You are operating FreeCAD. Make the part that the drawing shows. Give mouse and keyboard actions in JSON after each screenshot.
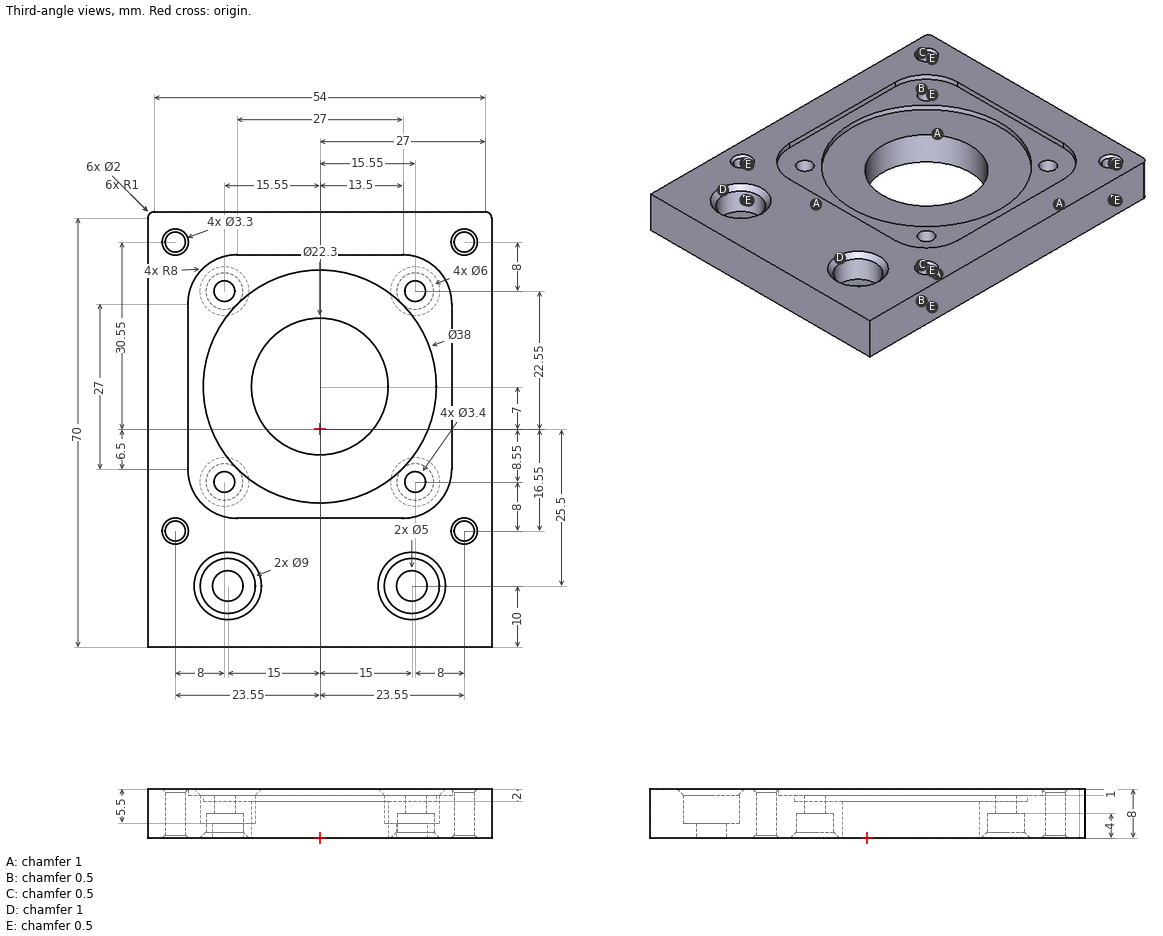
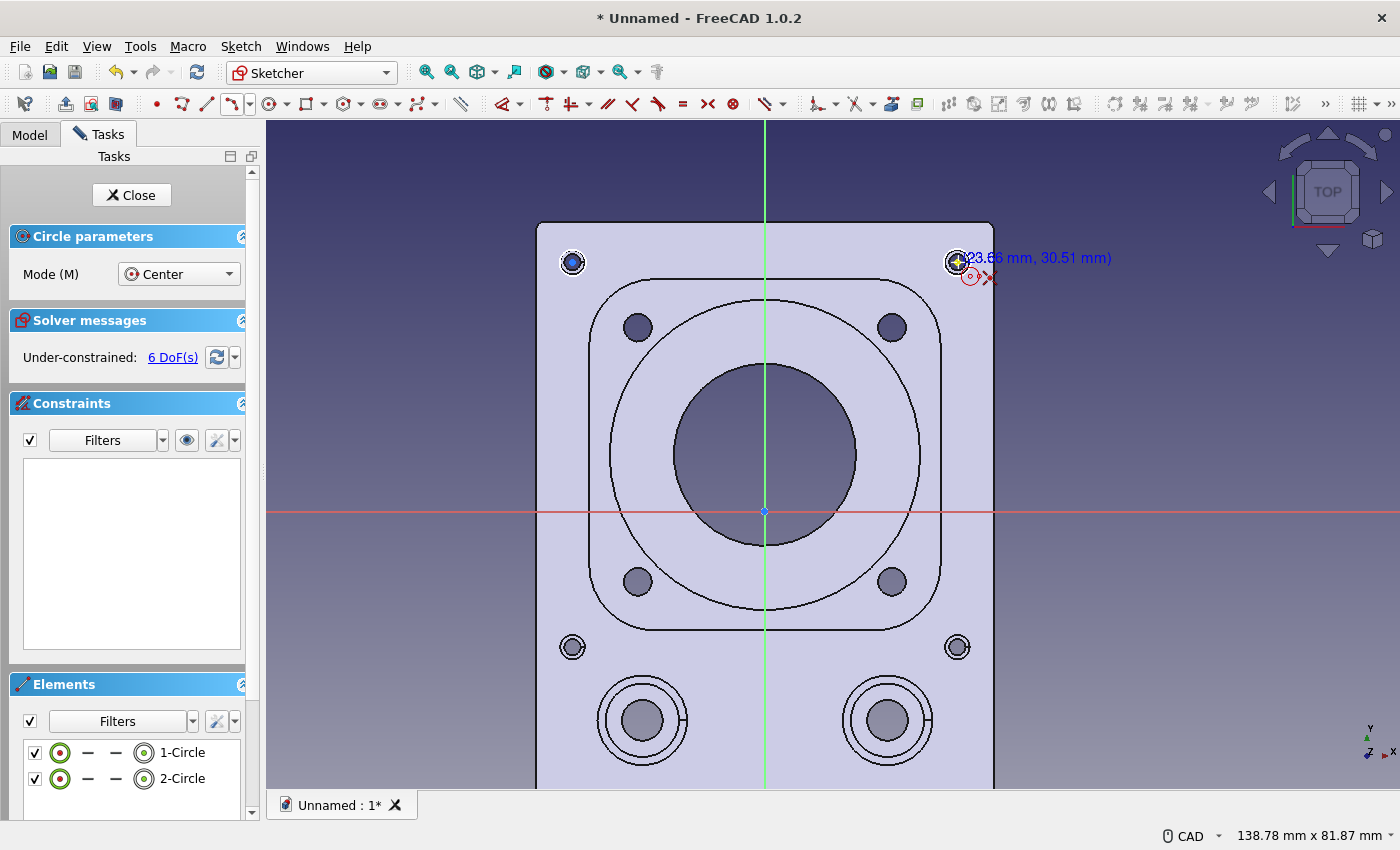
{"action": "scroll", "coordinate": [957, 647], "scroll_direction": "up", "scroll_amount": 3}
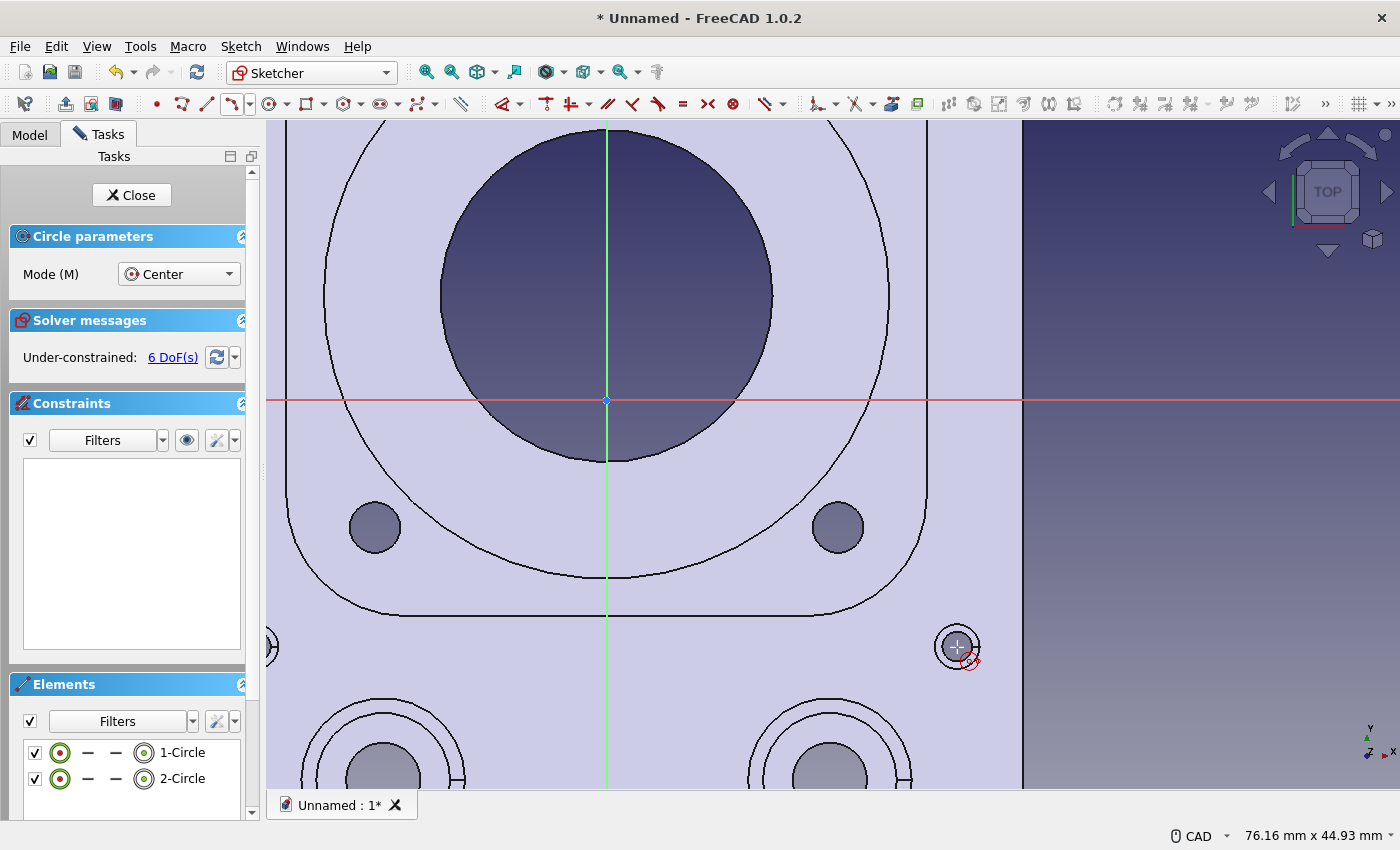
{"action": "left_click", "coordinate": [957, 647]}
{"action": "left_click", "coordinate": [975, 629]}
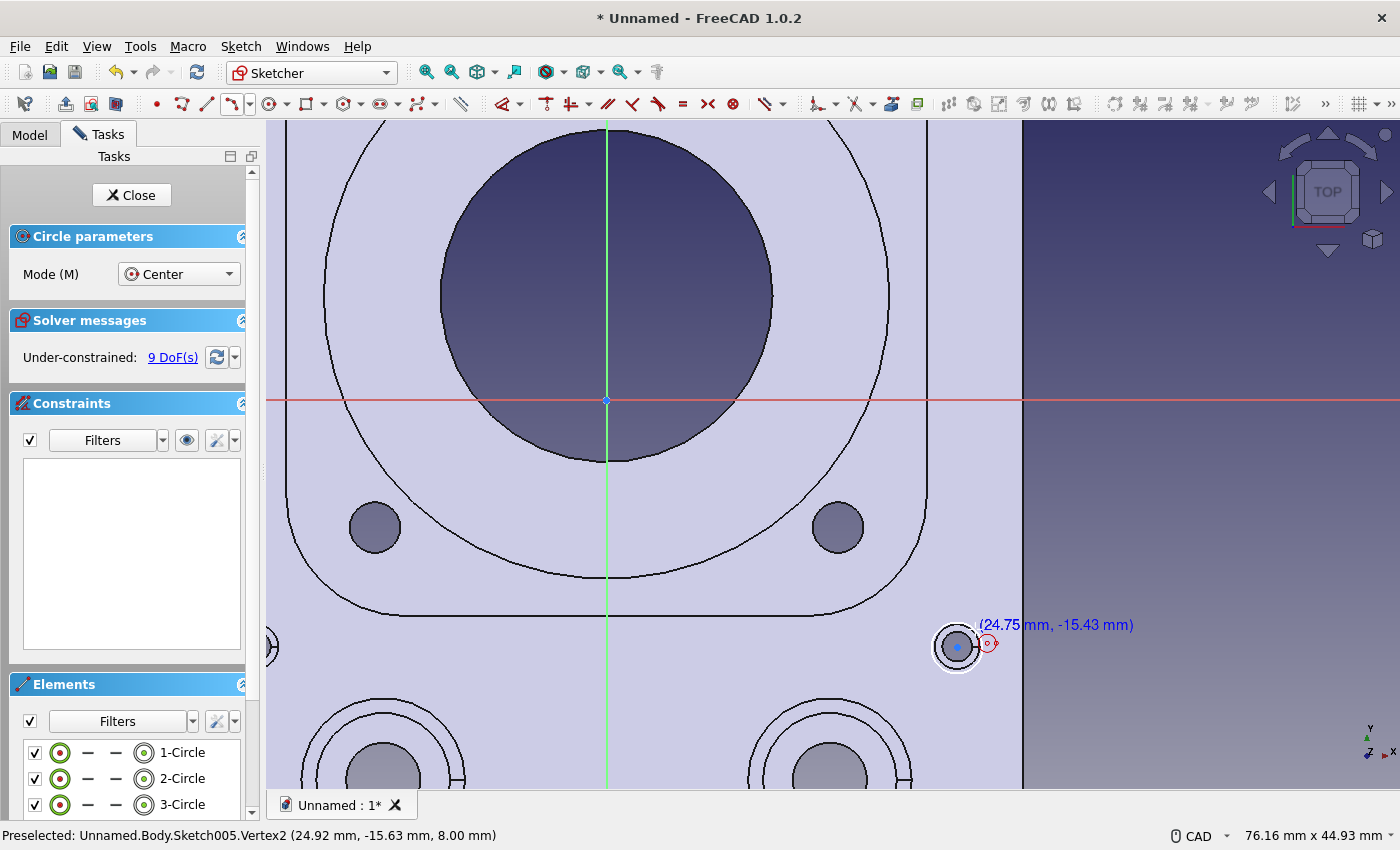
{"action": "scroll", "coordinate": [957, 647], "scroll_direction": "down", "scroll_amount": 3}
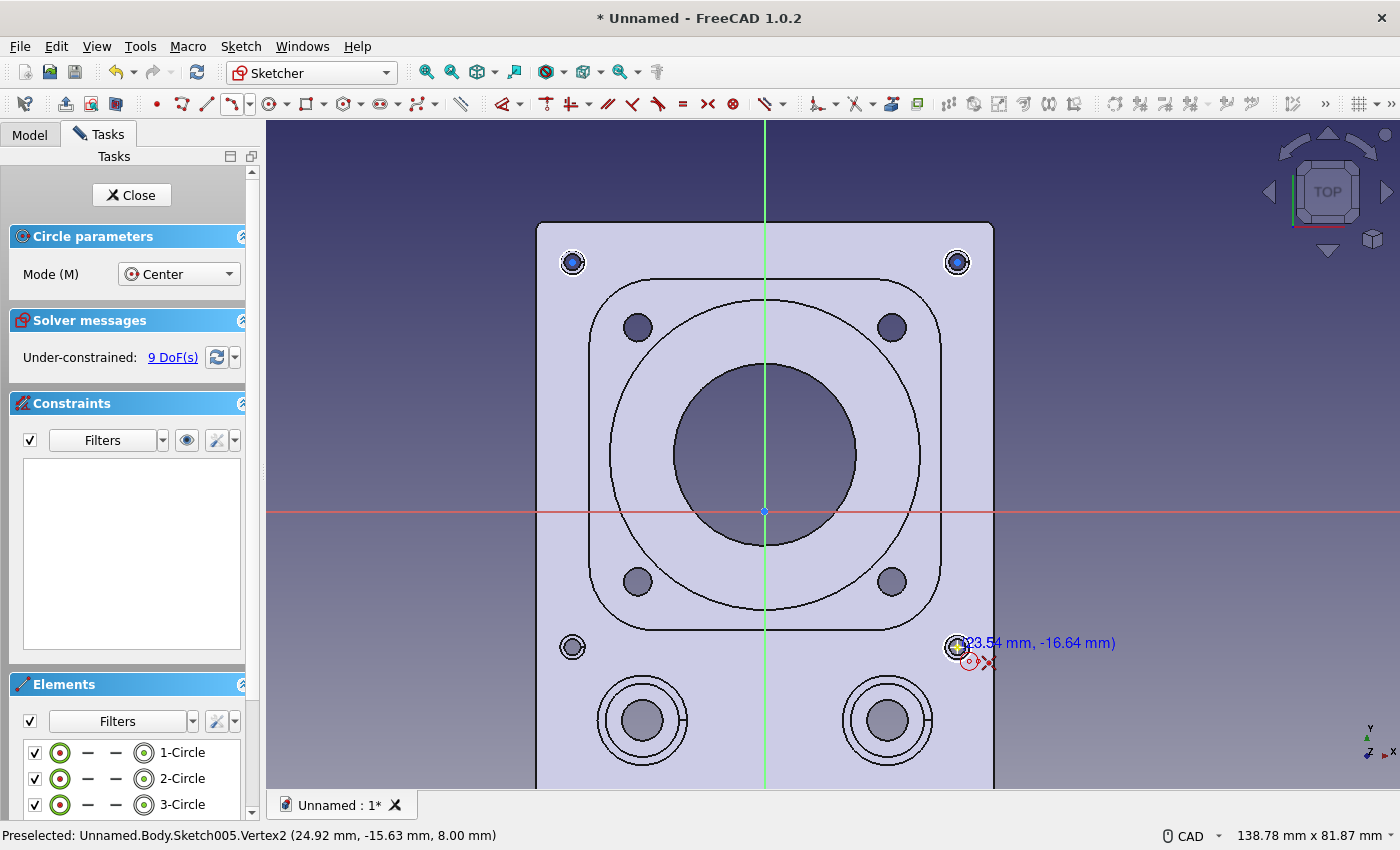
{"action": "scroll", "coordinate": [573, 647], "scroll_direction": "up", "scroll_amount": 3}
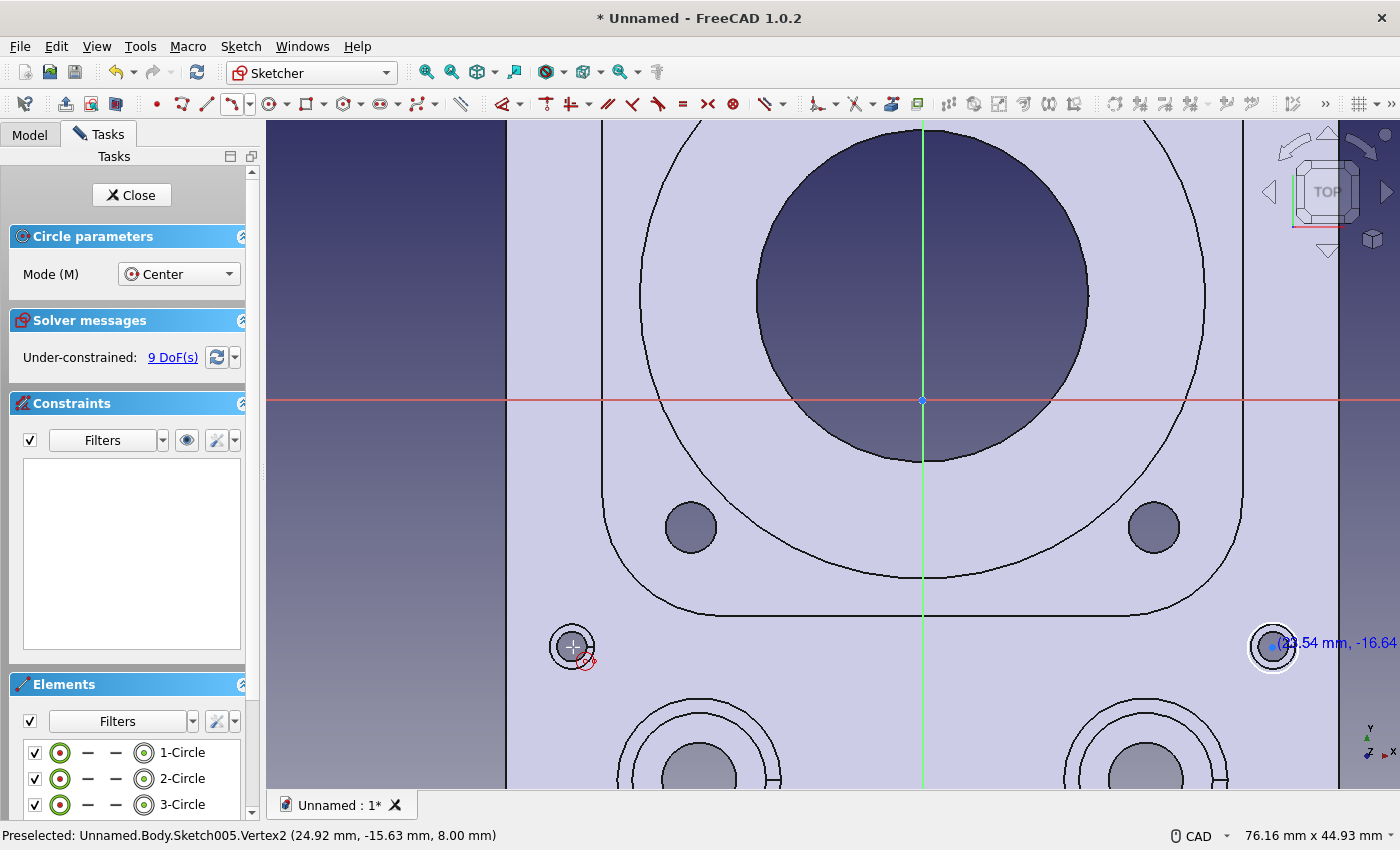
{"action": "left_click", "coordinate": [572, 647]}
{"action": "left_click", "coordinate": [589, 629]}
{"action": "key", "text": "Escape"}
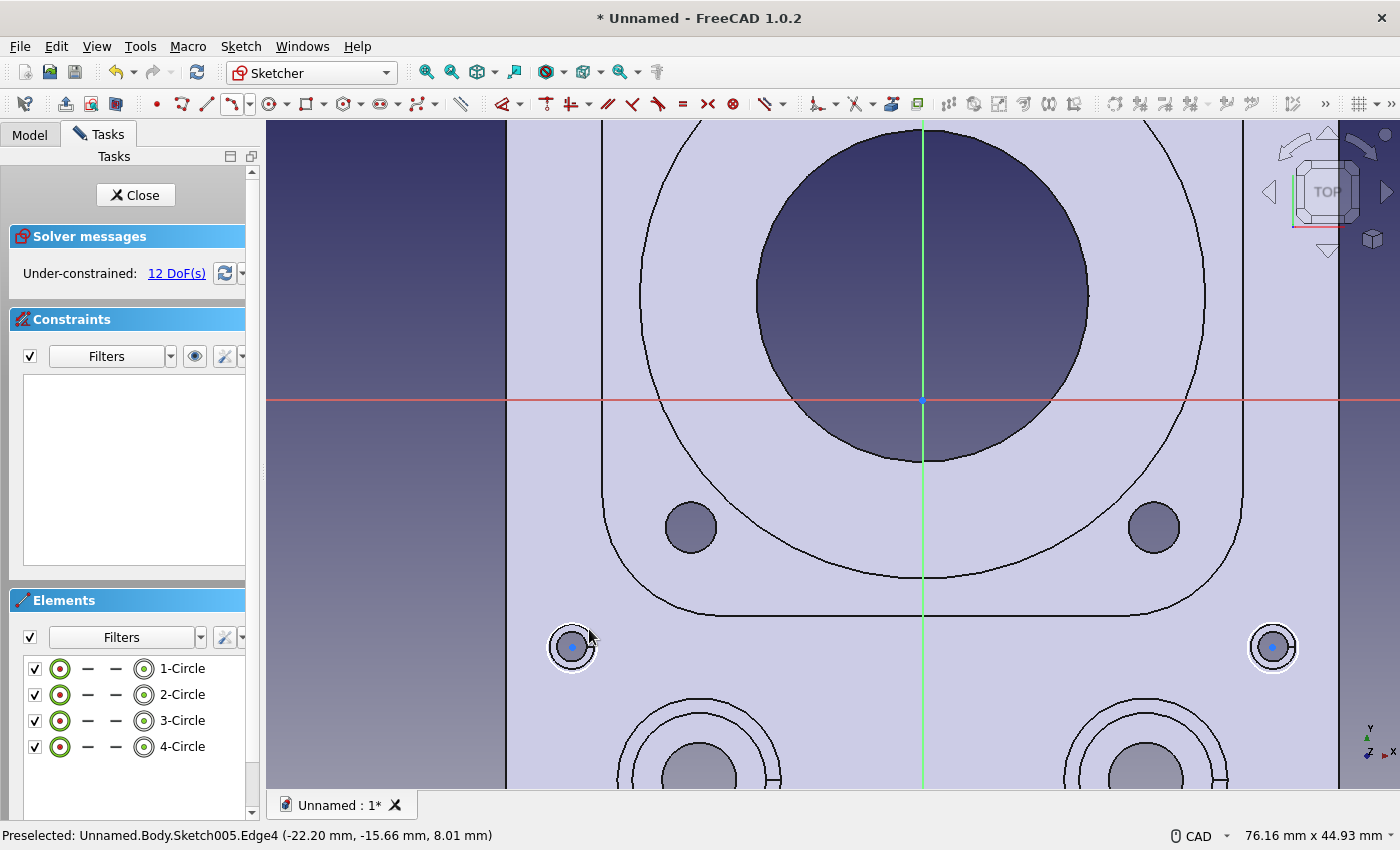
{"action": "scroll", "coordinate": [572, 647], "scroll_direction": "down", "scroll_amount": 3}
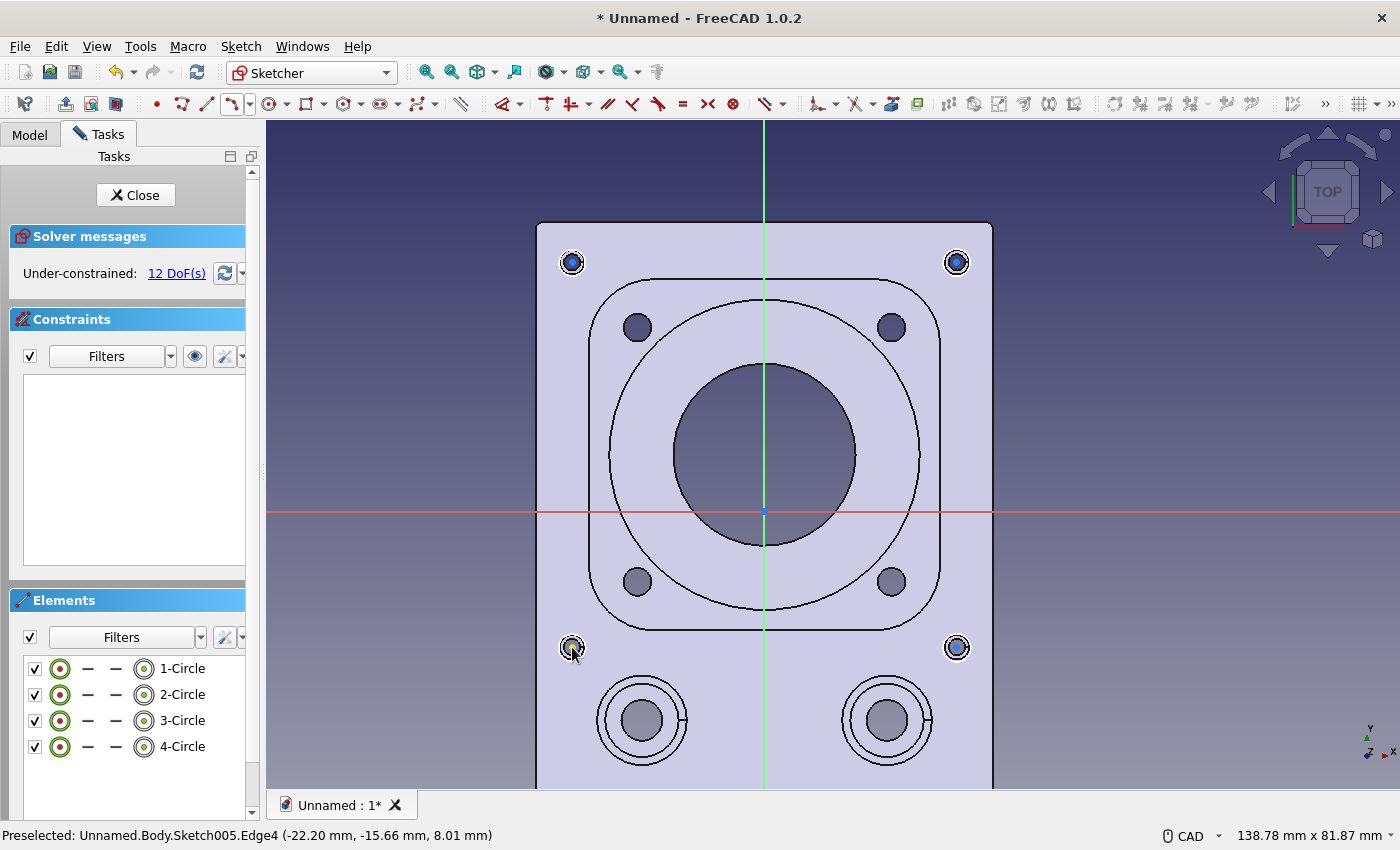
{"action": "left_click", "coordinate": [582, 253]}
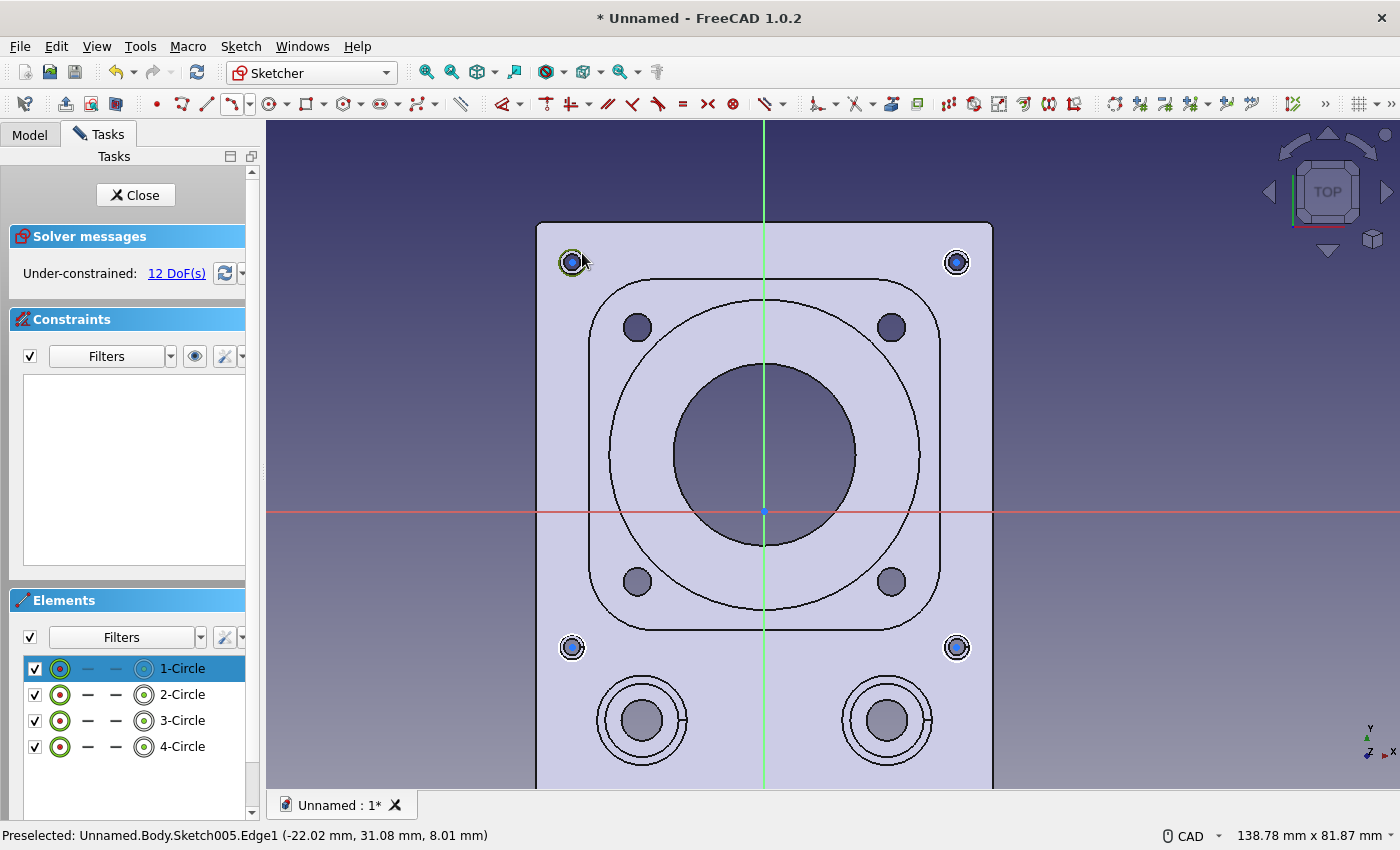
{"action": "left_click", "coordinate": [966, 253]}